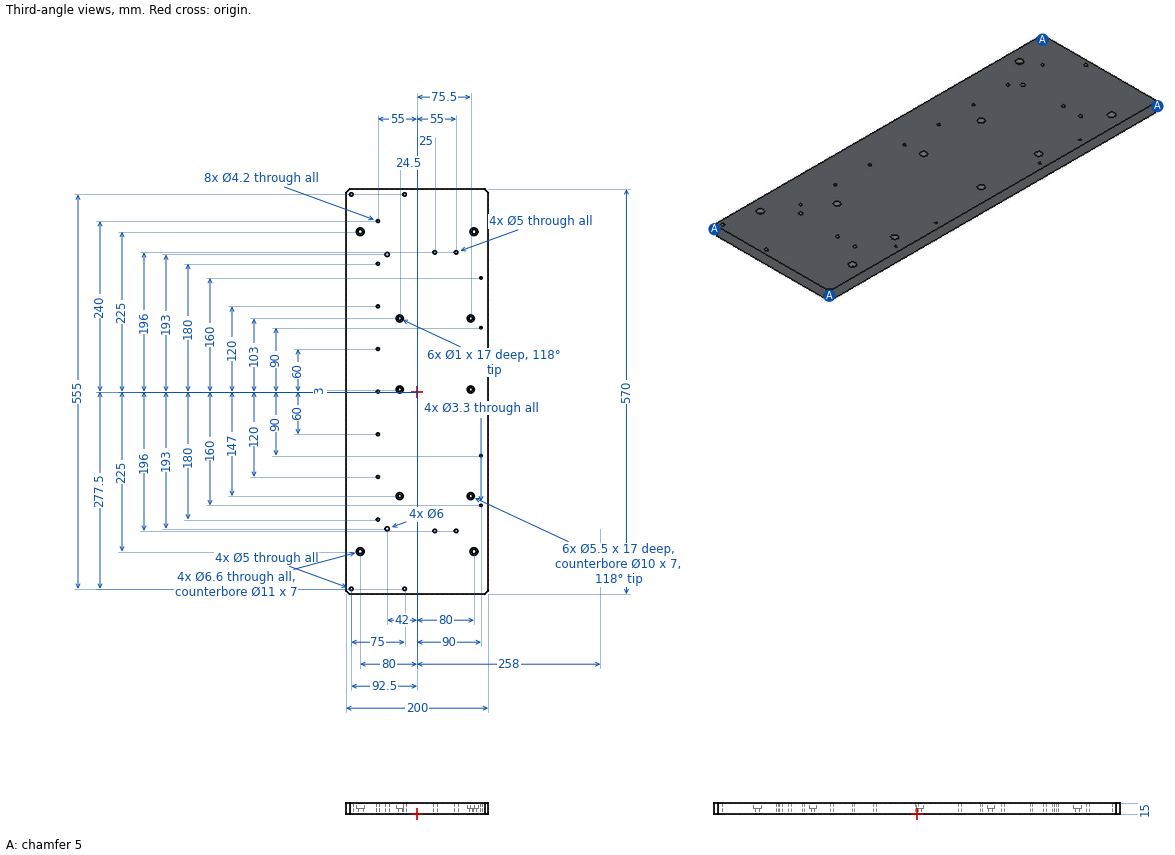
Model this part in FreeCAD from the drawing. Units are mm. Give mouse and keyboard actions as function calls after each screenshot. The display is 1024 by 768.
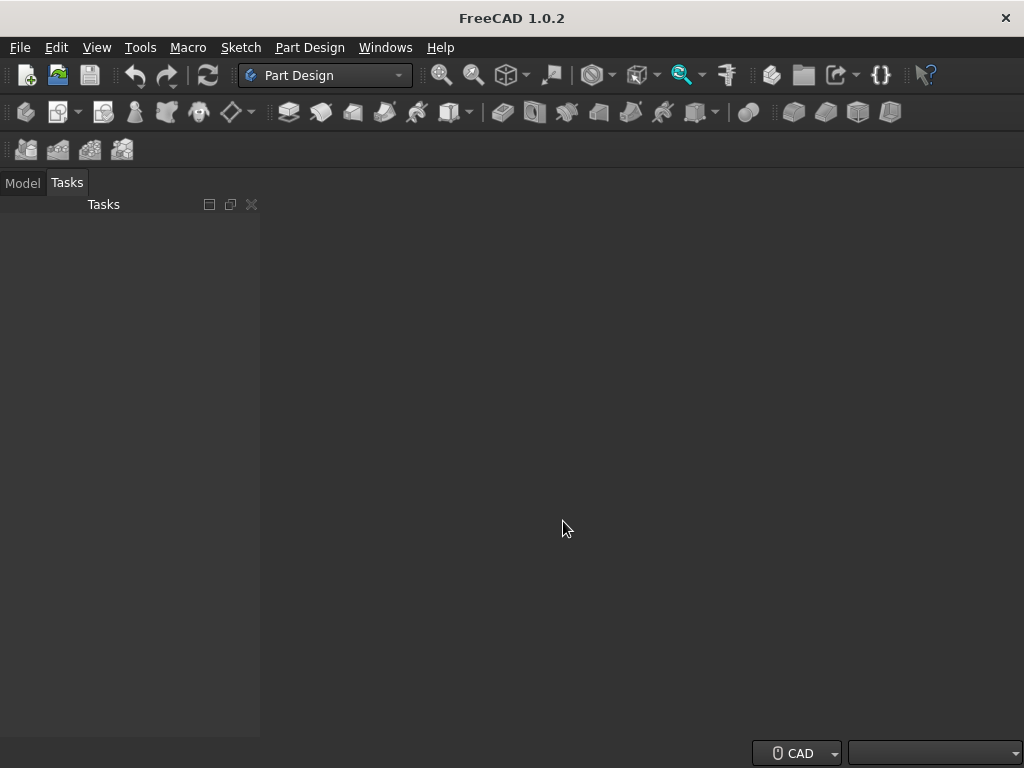
click(26, 76)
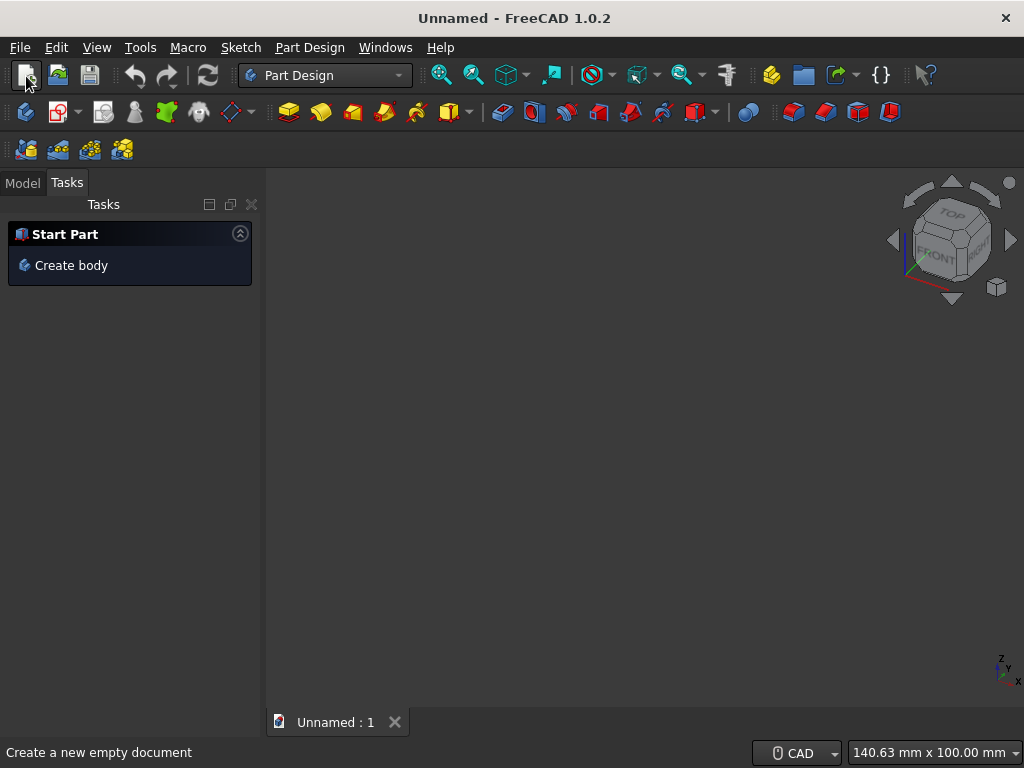
click(58, 112)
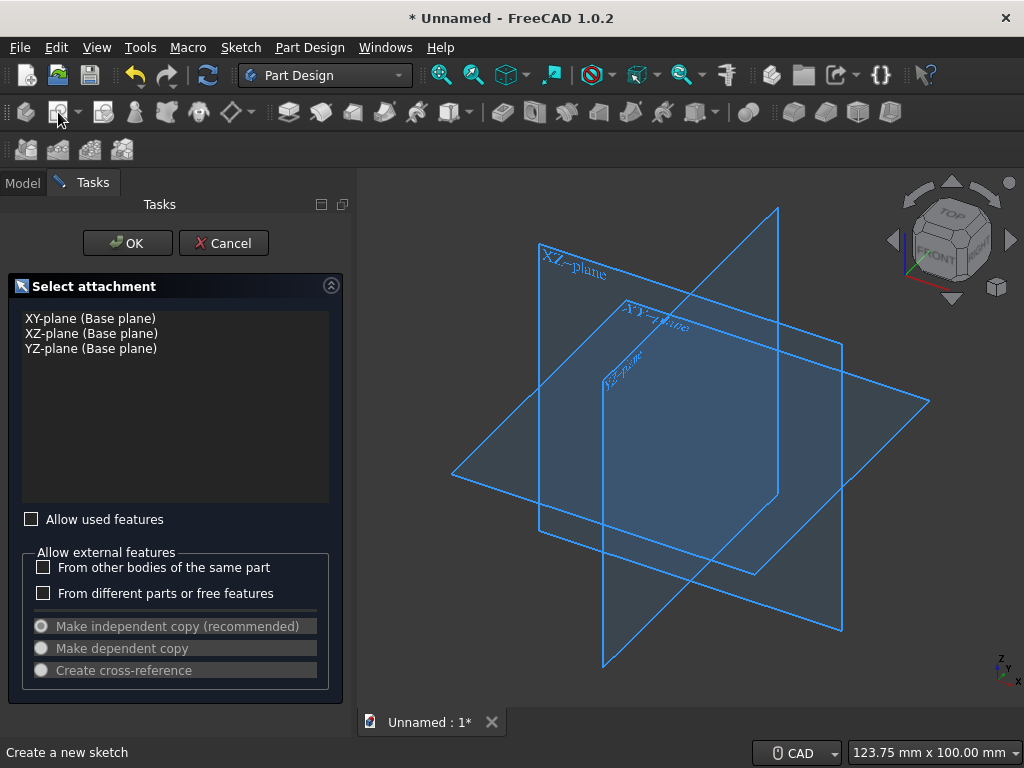
click(82, 318)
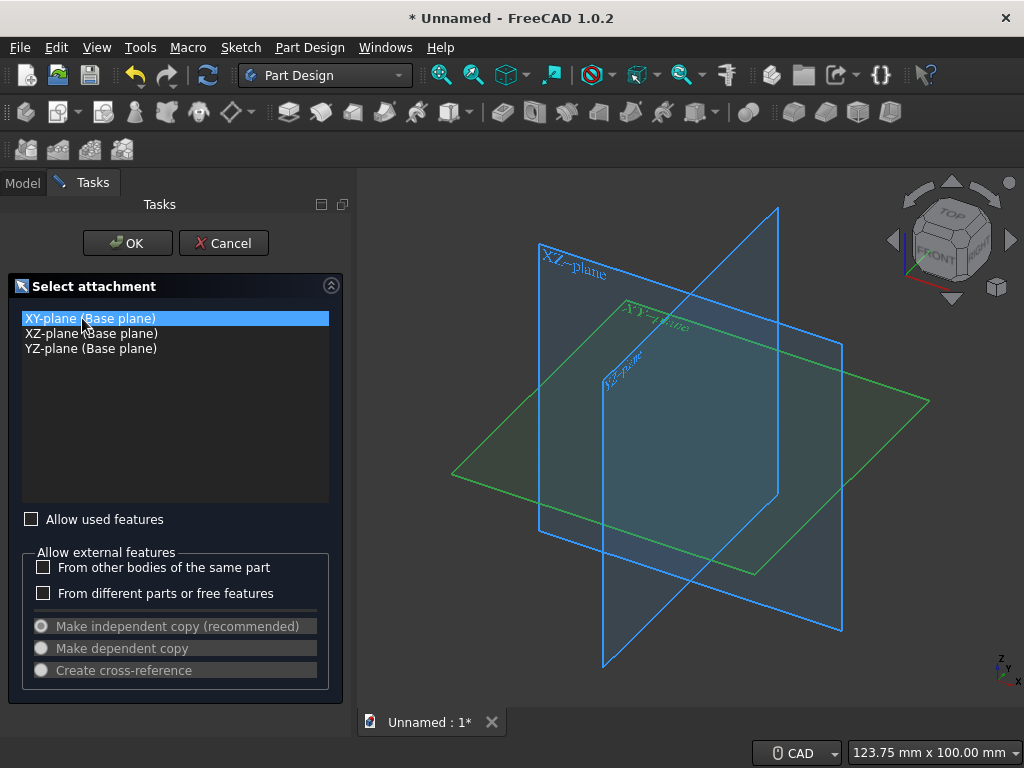
click(128, 243)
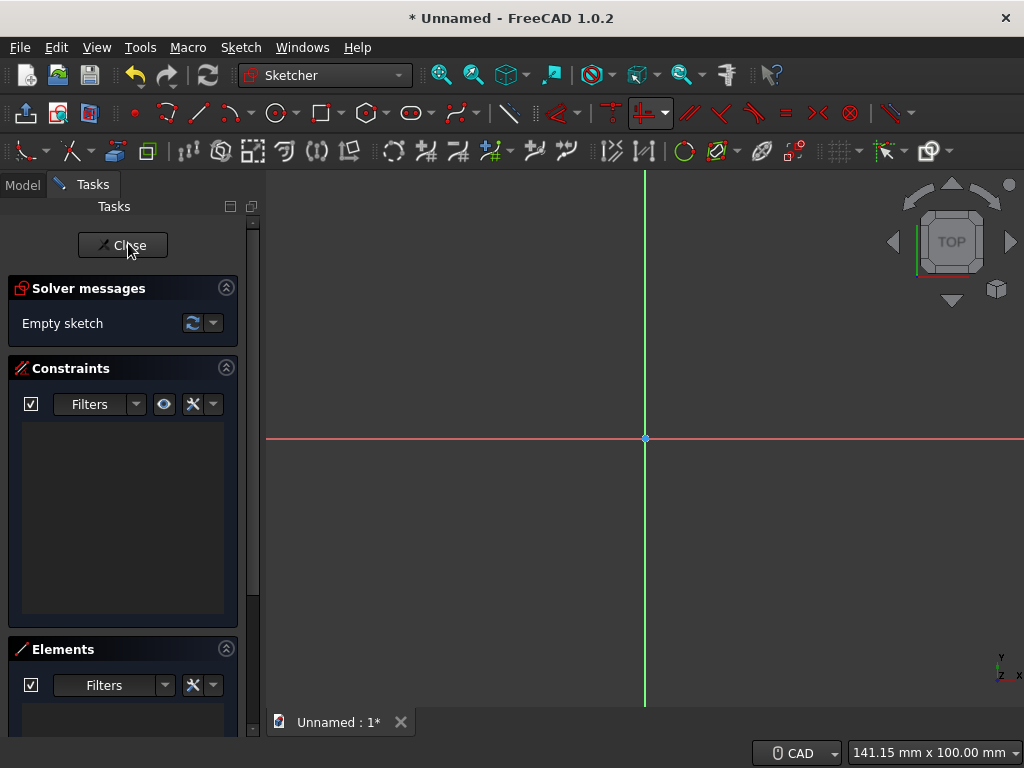
scroll(568, 439, down, 11)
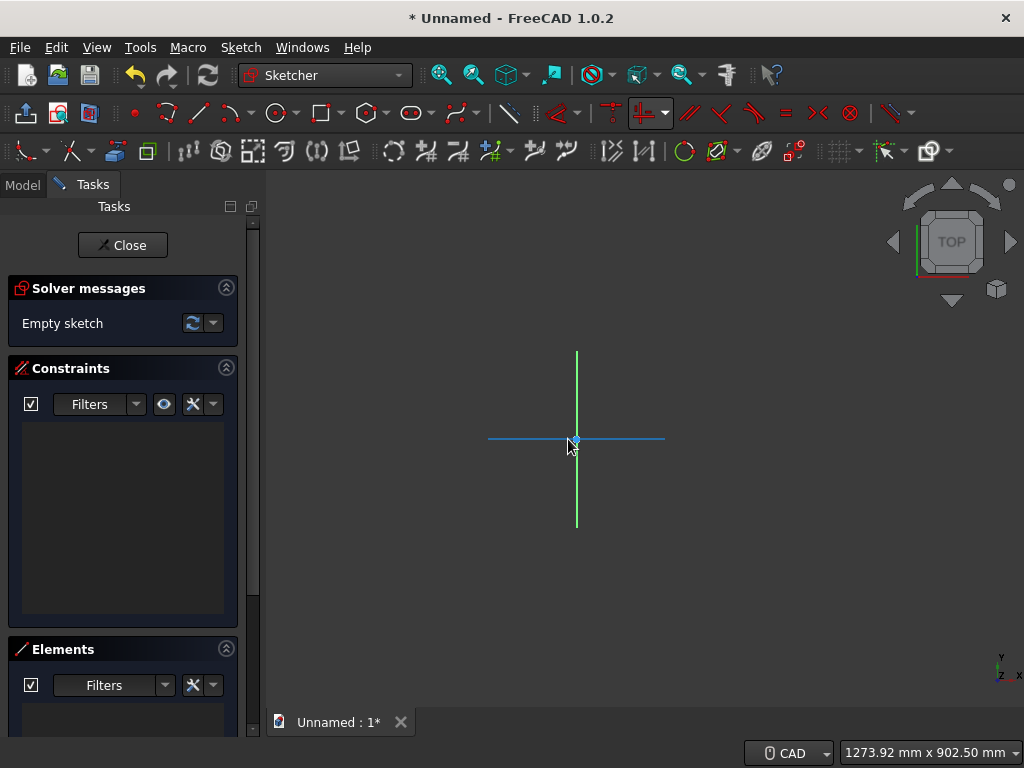
key(g)
key(v)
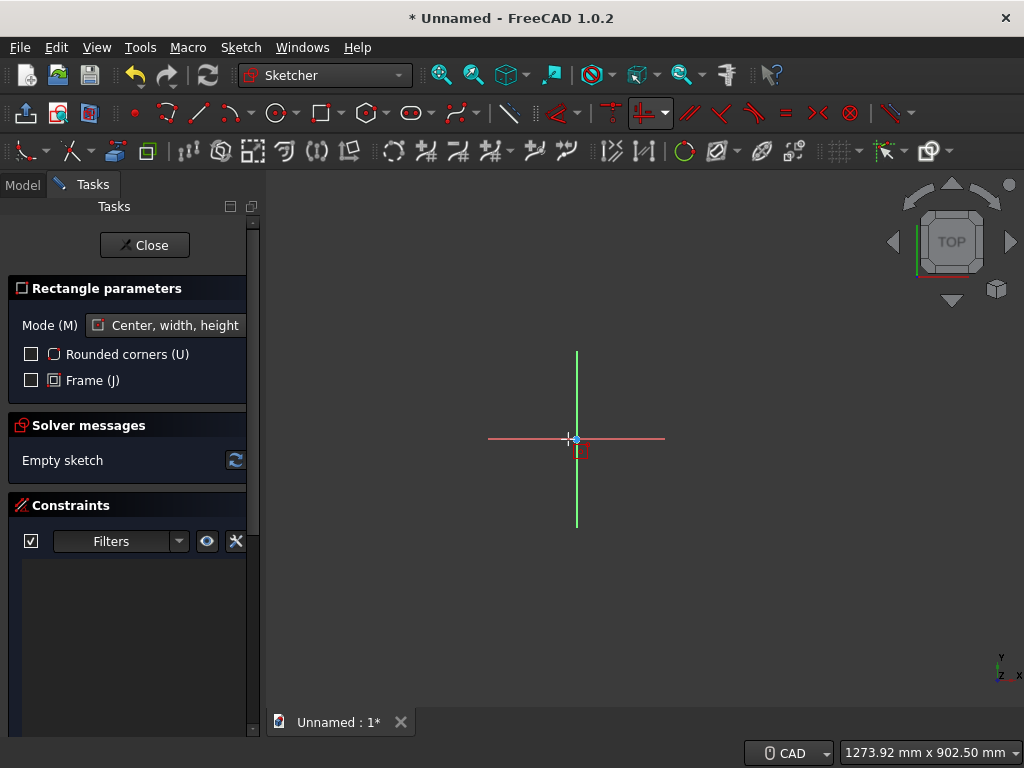
click(577, 439)
move(636, 270)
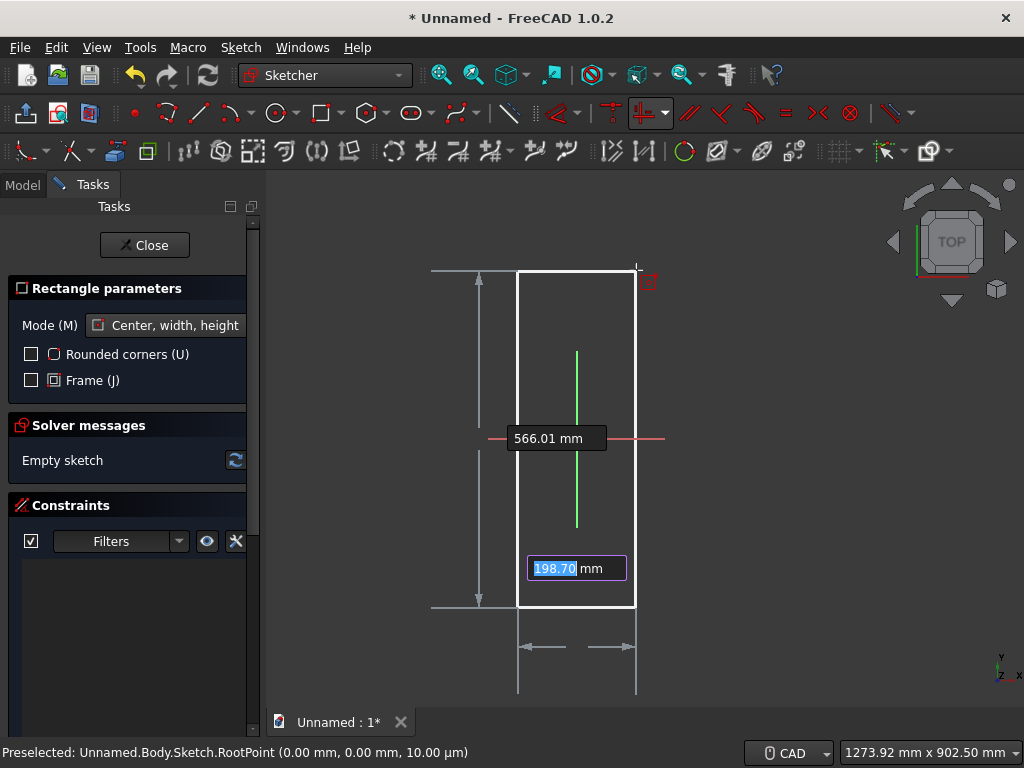
text(200)
key(Tab)
text(570)
key(Return)
key(Escape)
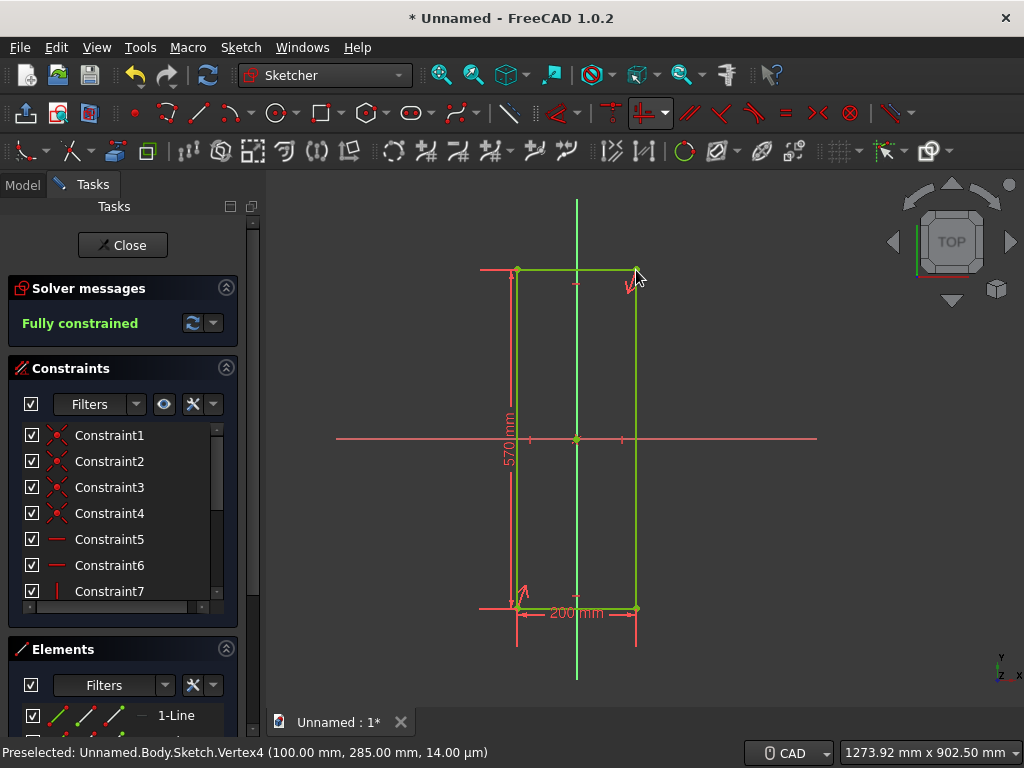
click(123, 245)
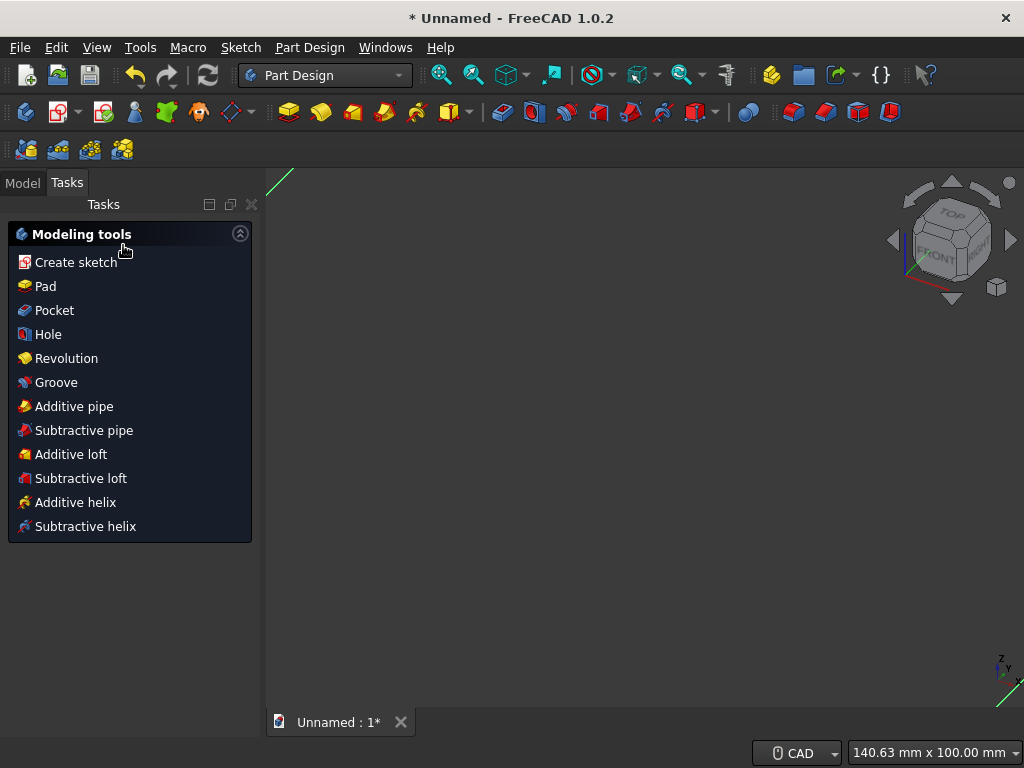
click(290, 112)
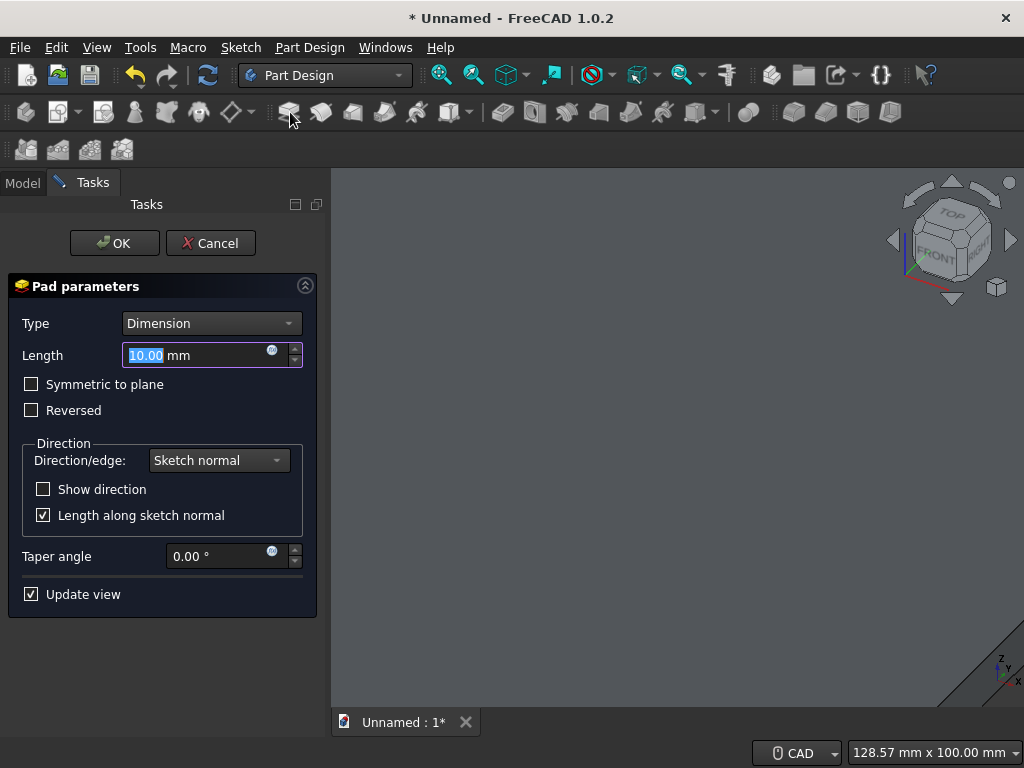
text(15)
key(Tab)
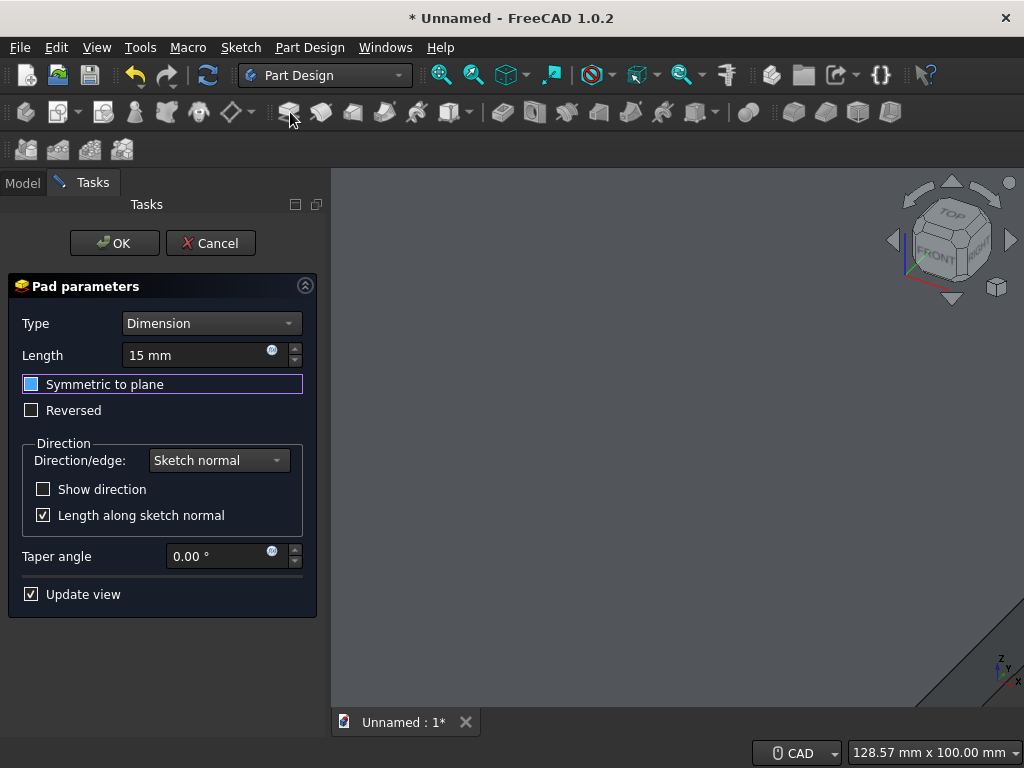
click(115, 243)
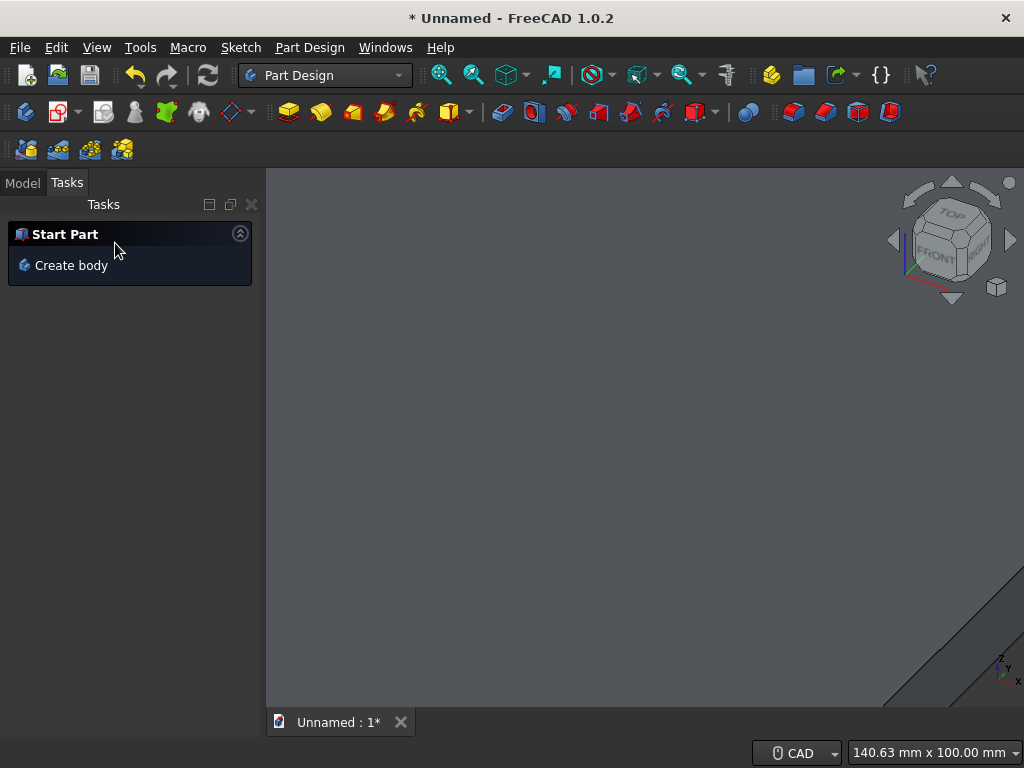
click(442, 76)